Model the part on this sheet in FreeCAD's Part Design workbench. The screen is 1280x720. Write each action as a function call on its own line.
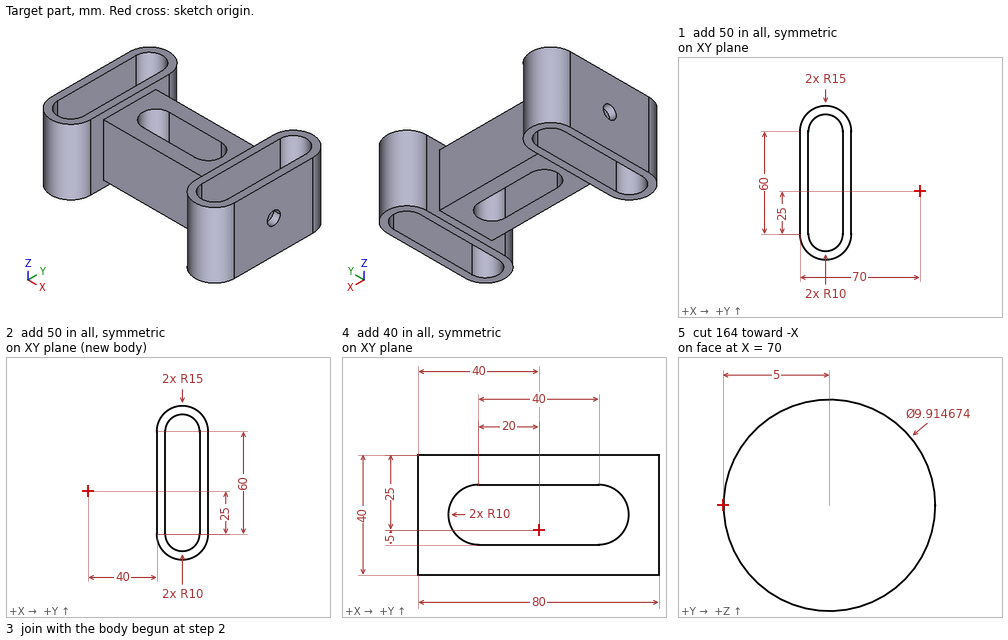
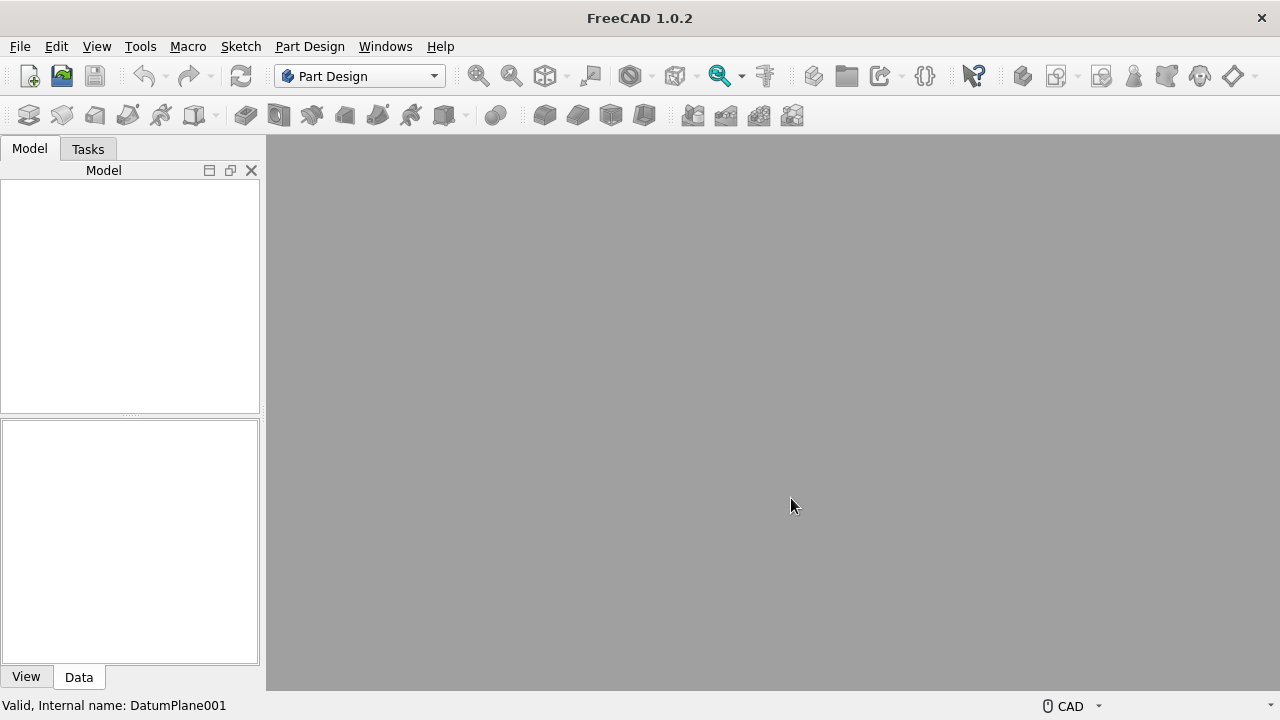
click(29, 76)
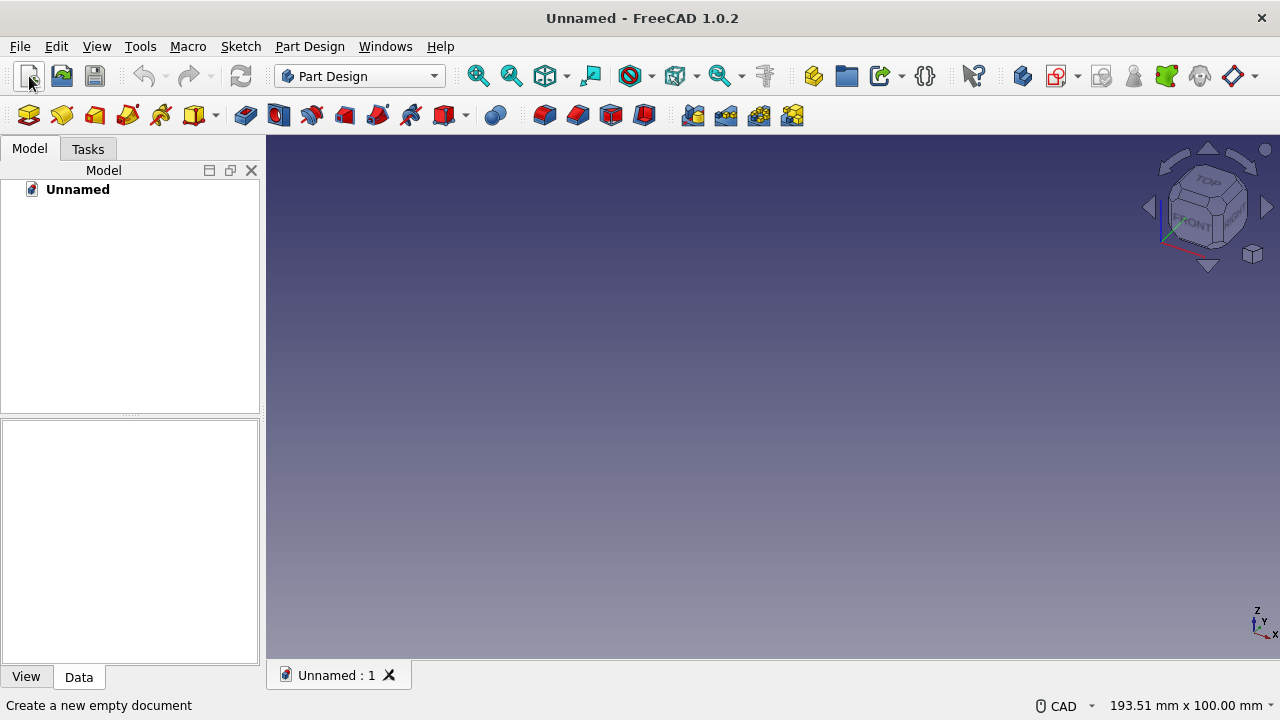
click(1056, 76)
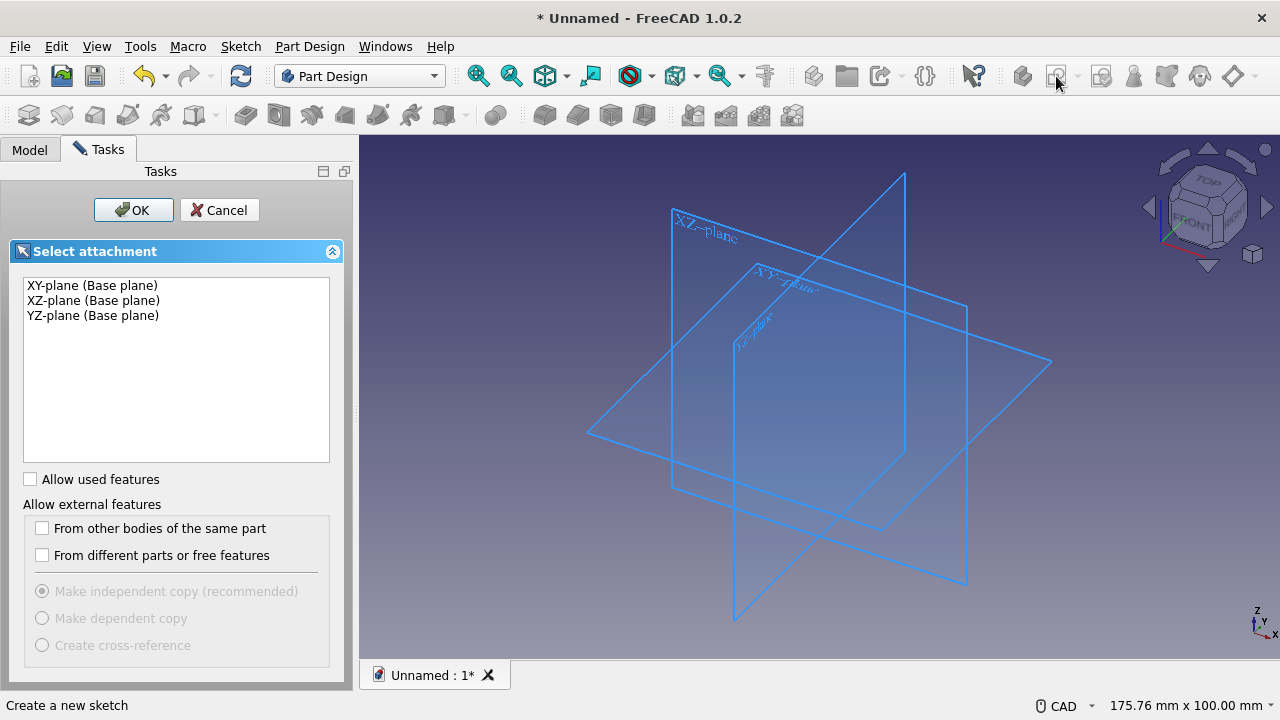
click(84, 286)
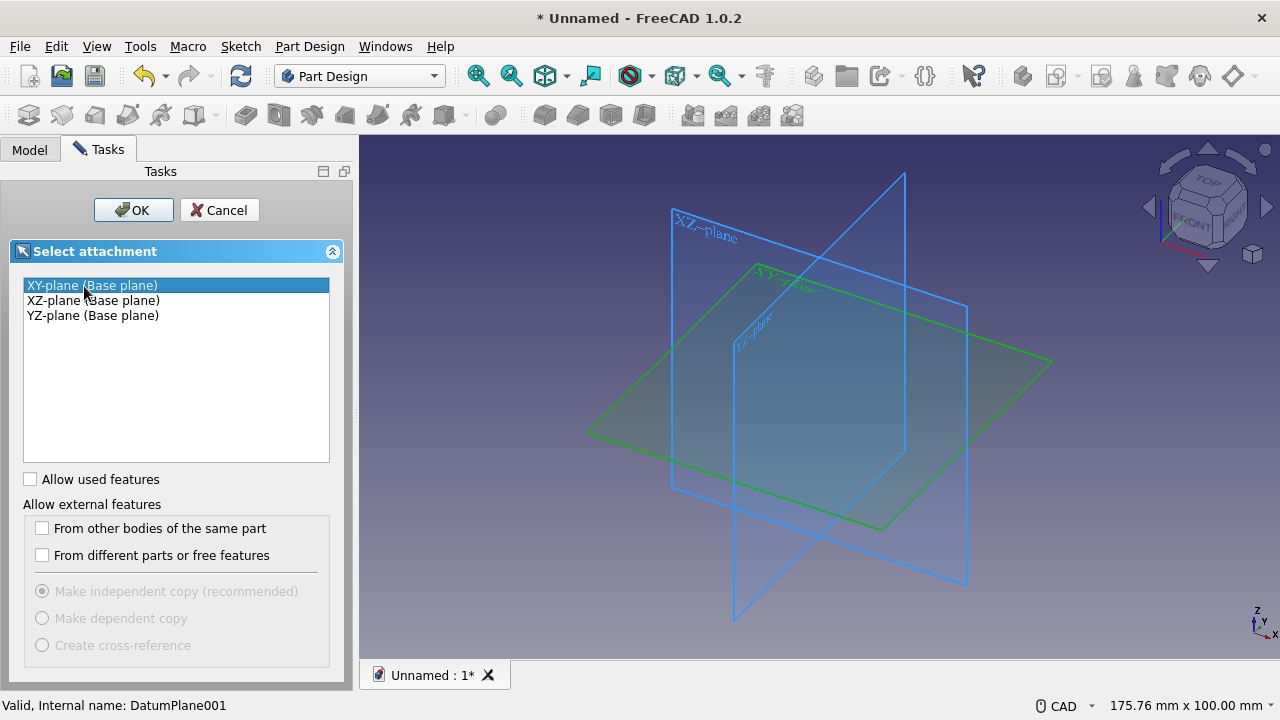
click(134, 210)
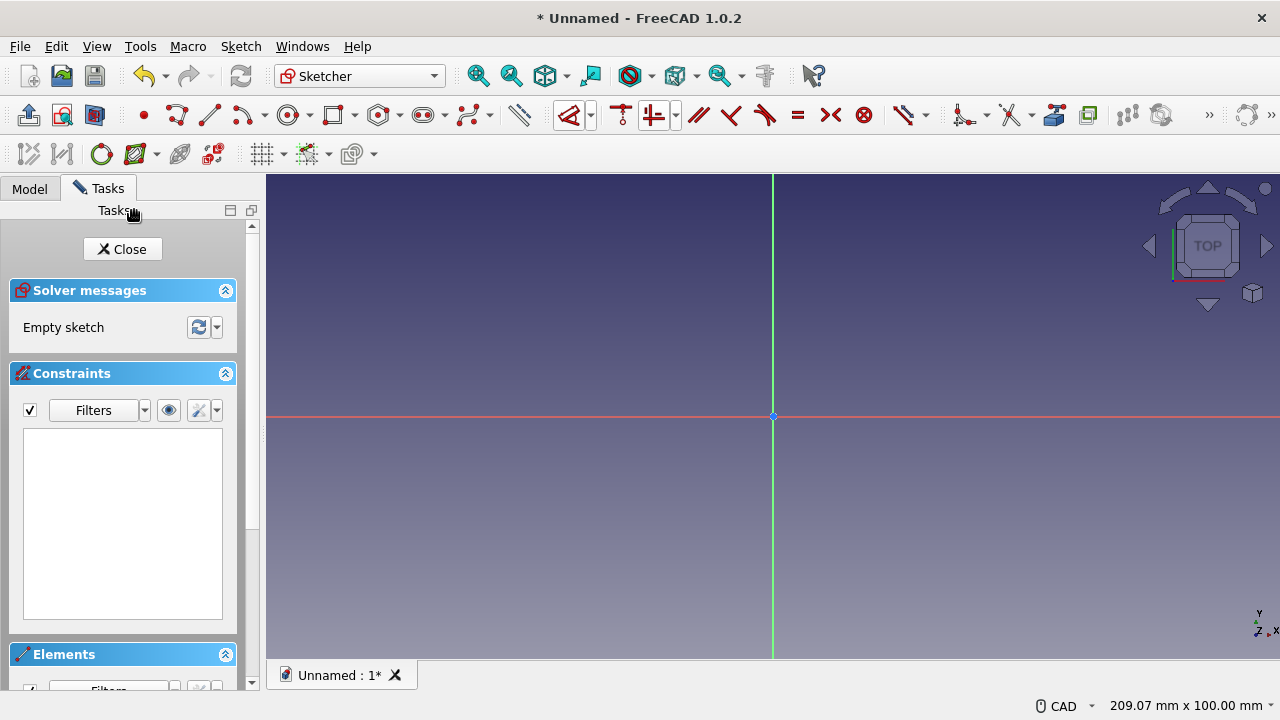
scroll(910, 466, down, 2)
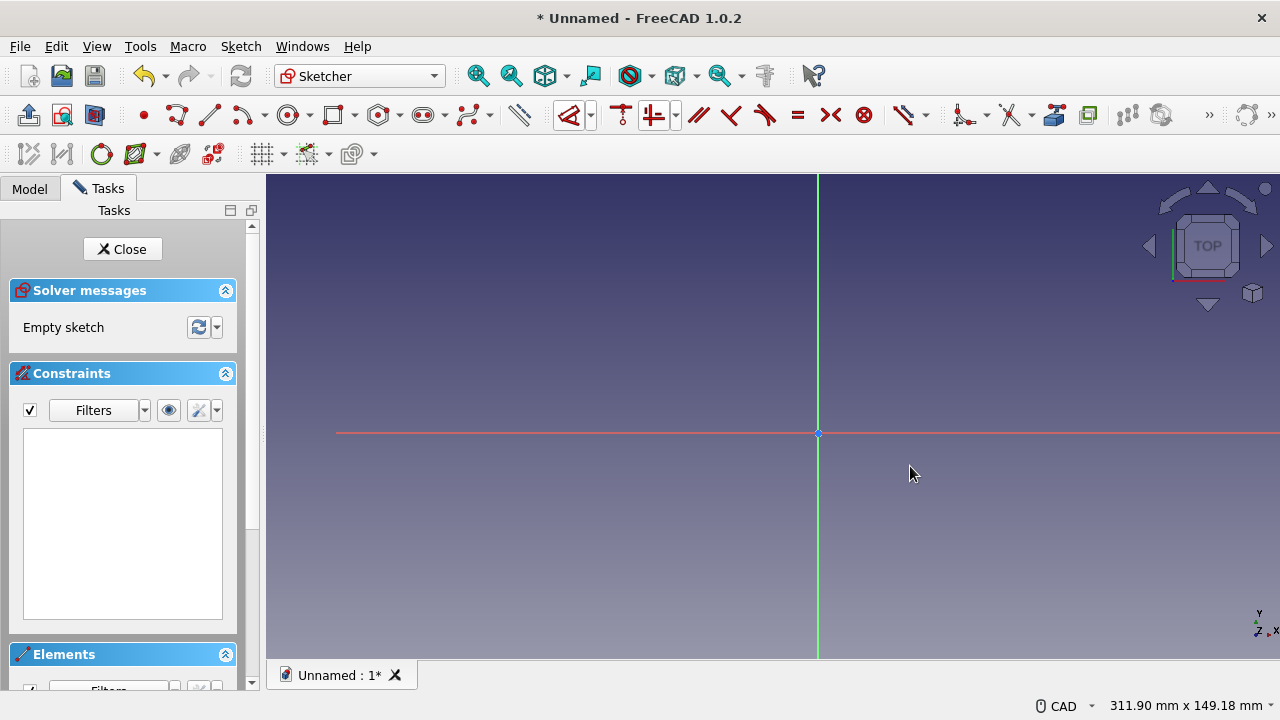
click(422, 116)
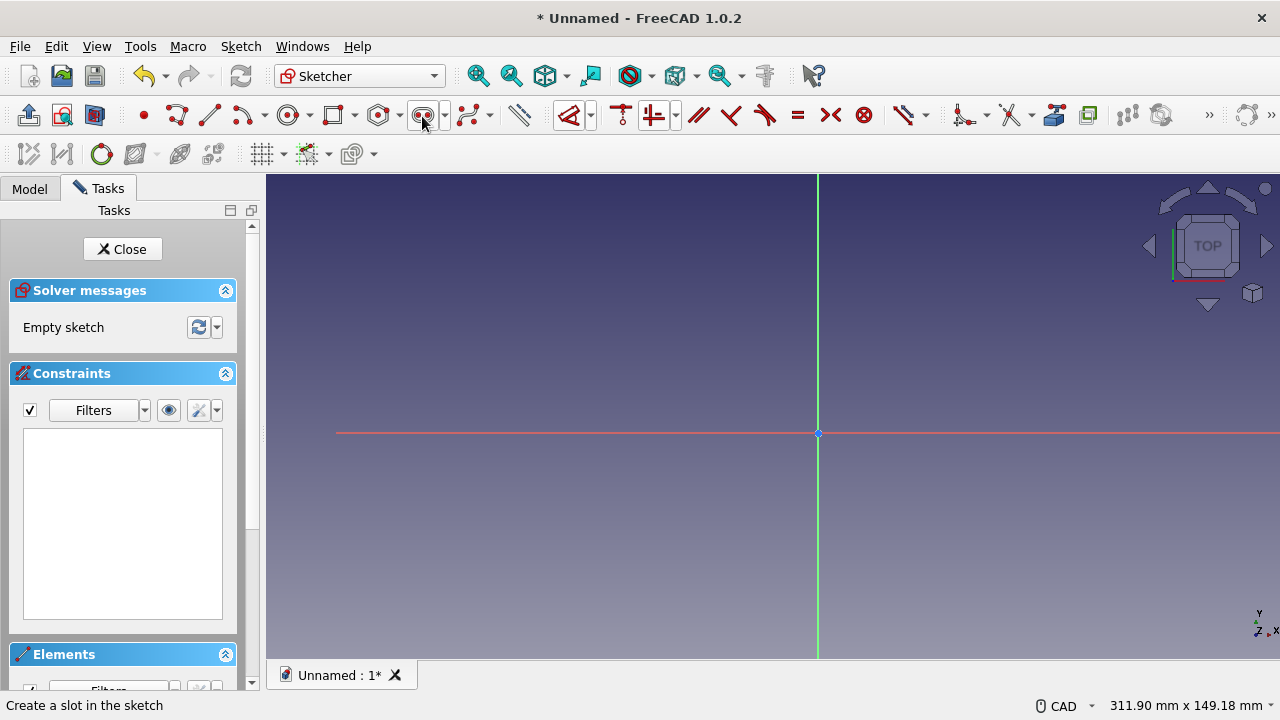
click(640, 514)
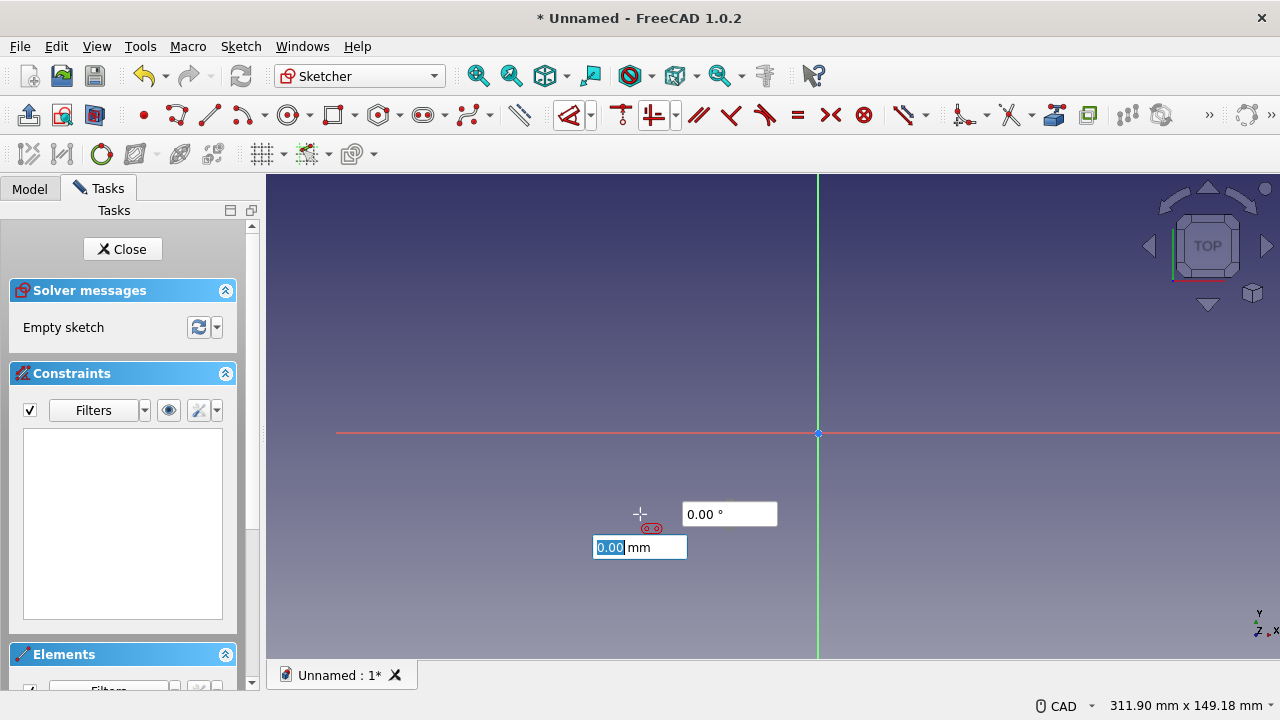
click(640, 319)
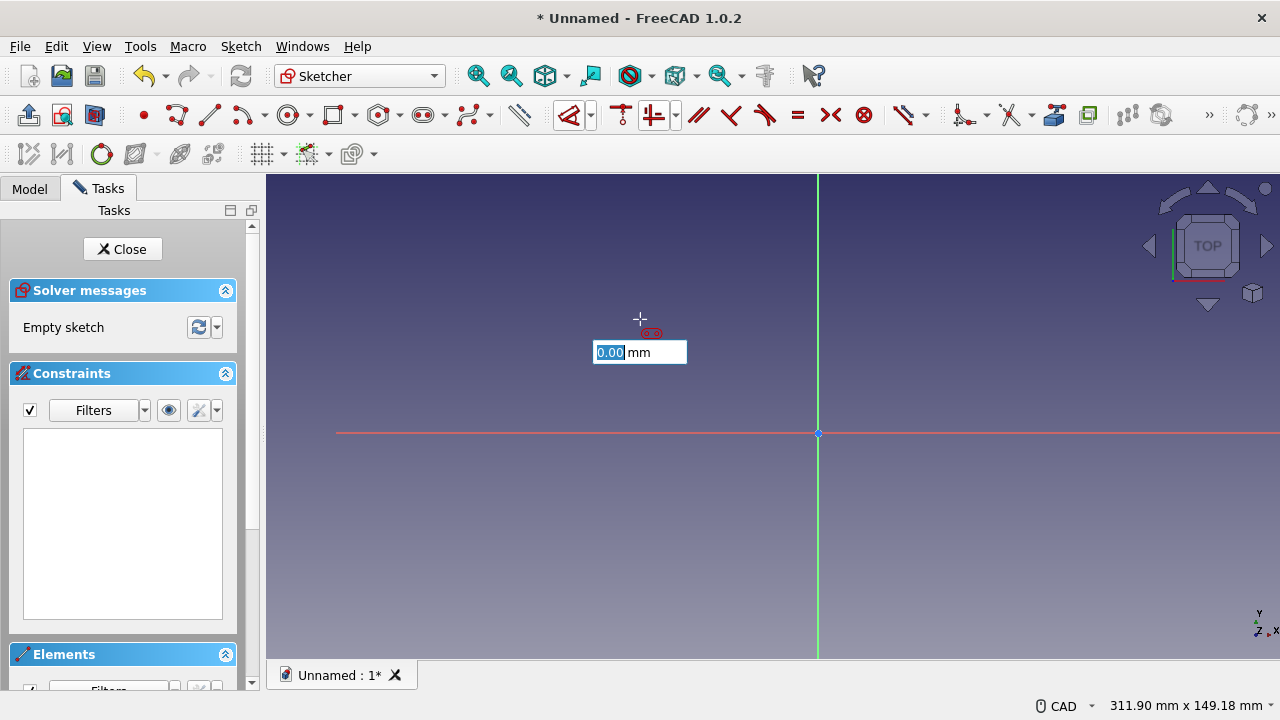
click(688, 417)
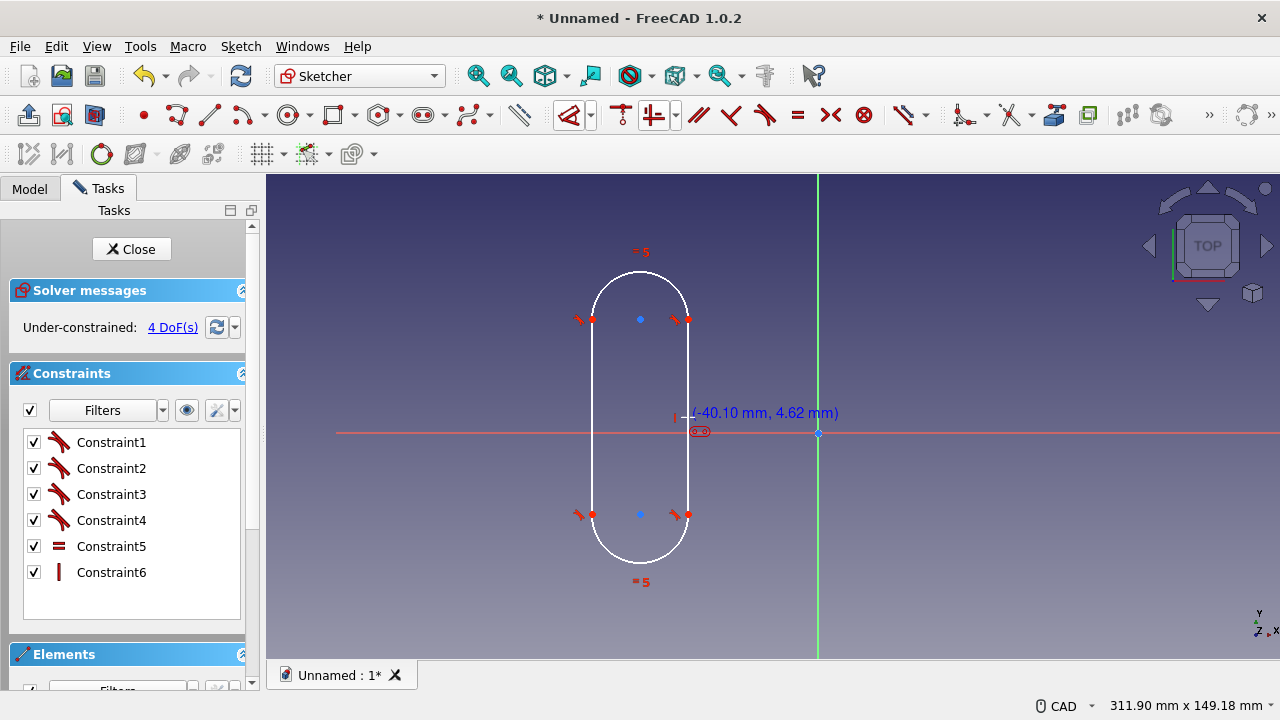
click(640, 515)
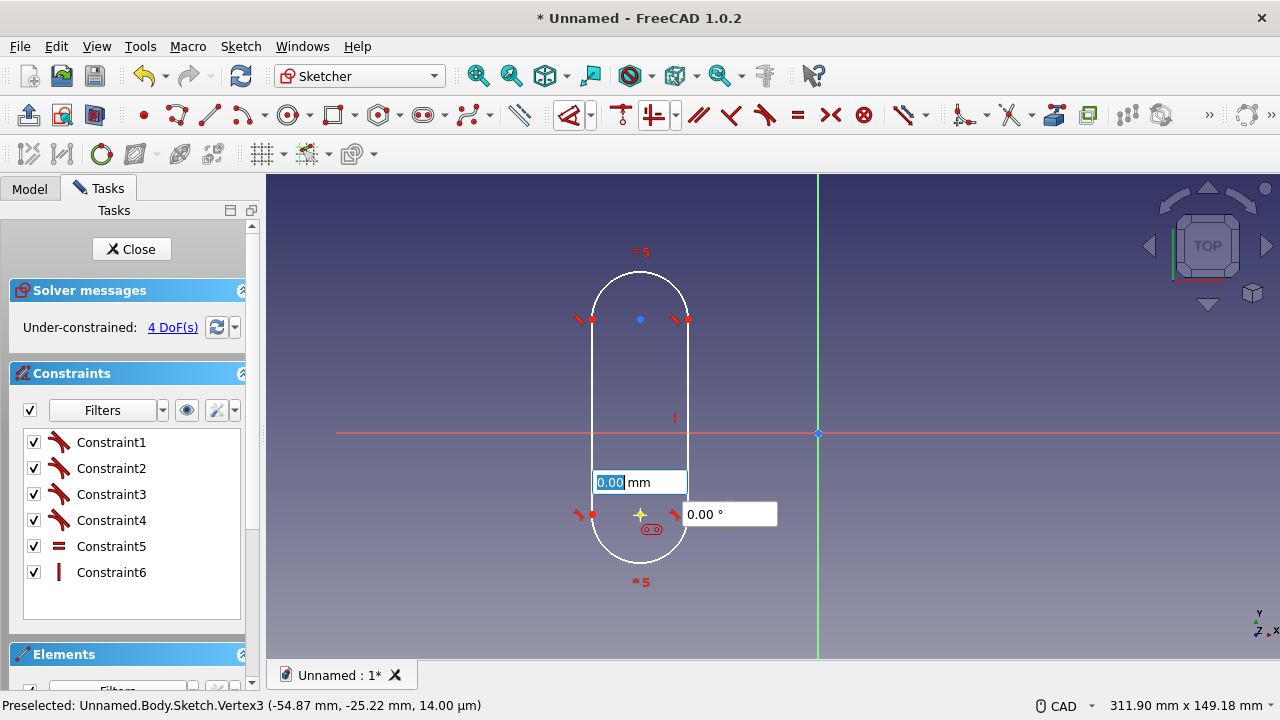
click(640, 320)